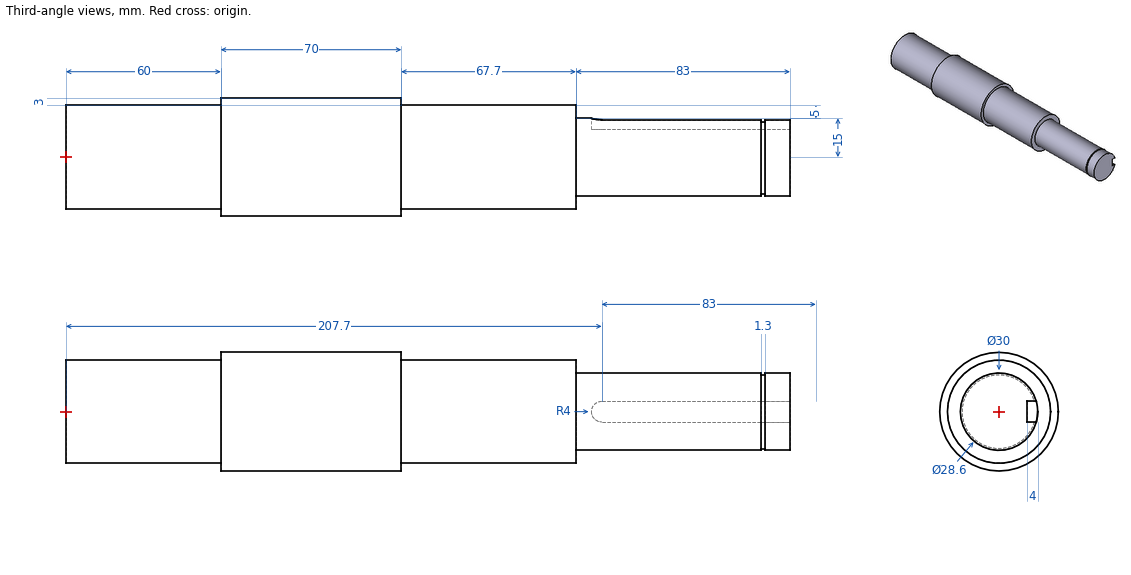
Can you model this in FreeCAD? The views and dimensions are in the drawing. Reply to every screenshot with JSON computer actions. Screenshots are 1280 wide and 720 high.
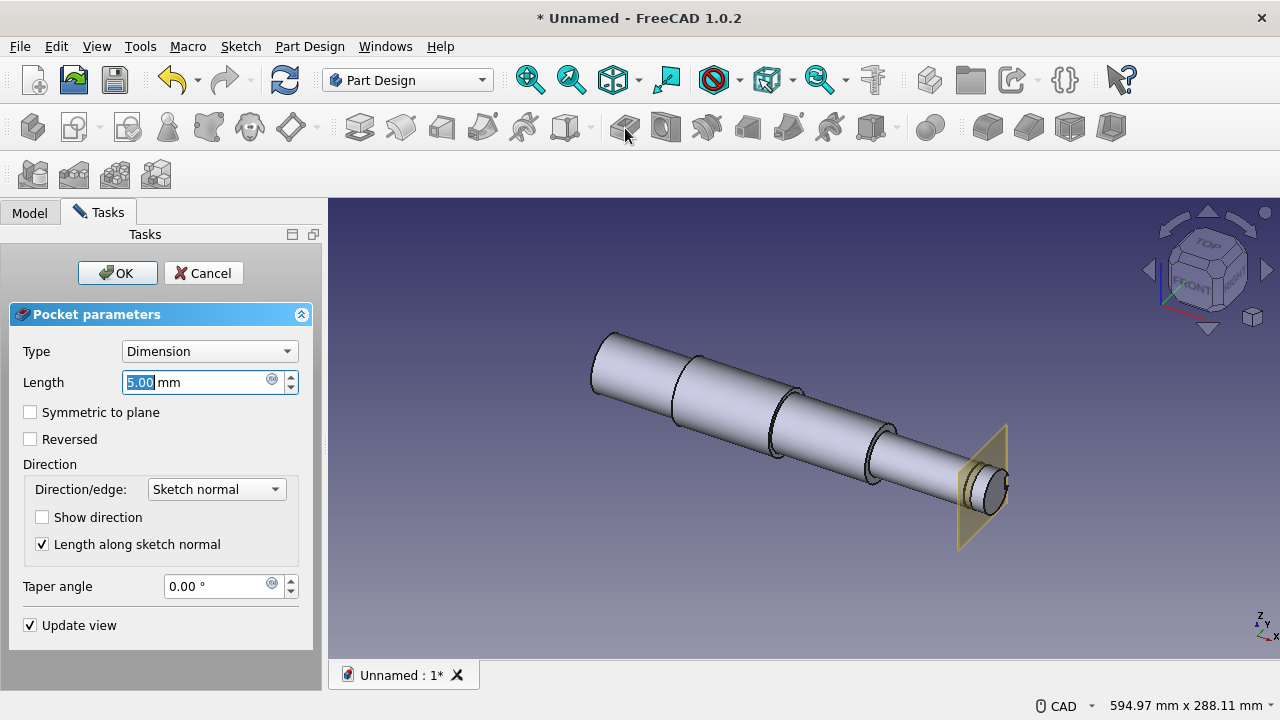
{"action": "type", "text": "1.3"}
{"action": "key", "text": "Tab"}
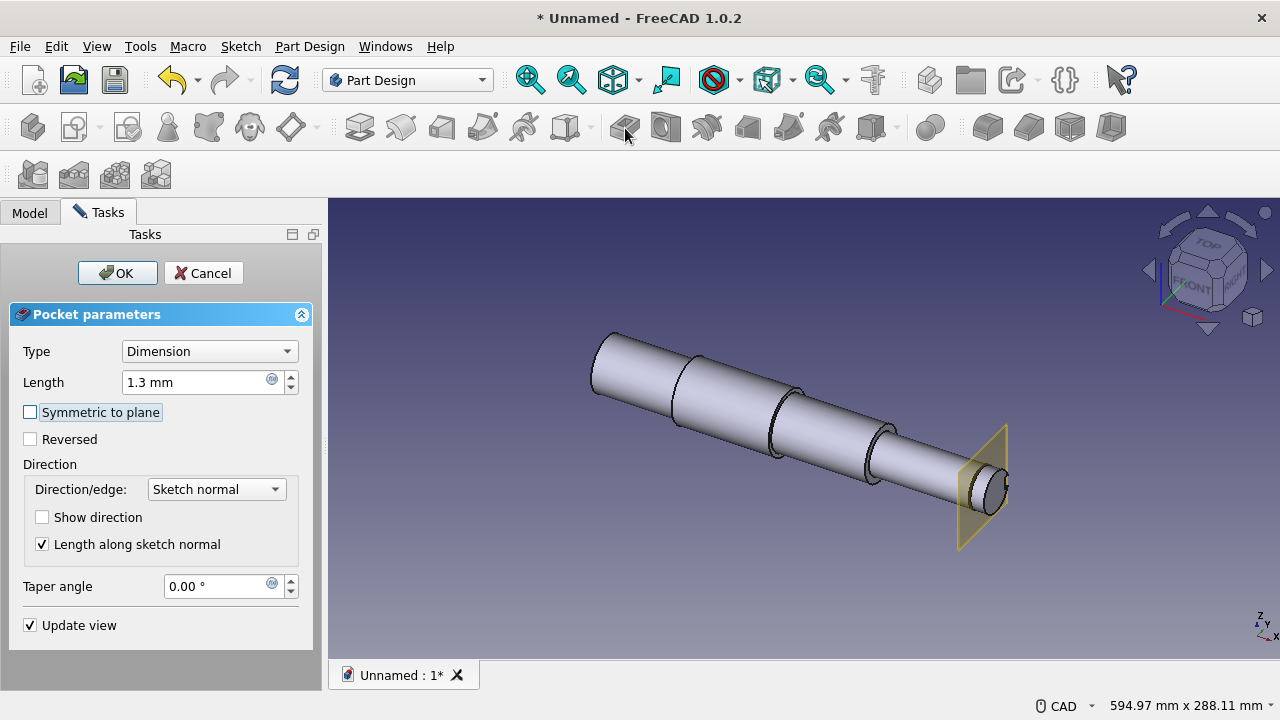
{"action": "left_click", "coordinate": [118, 273]}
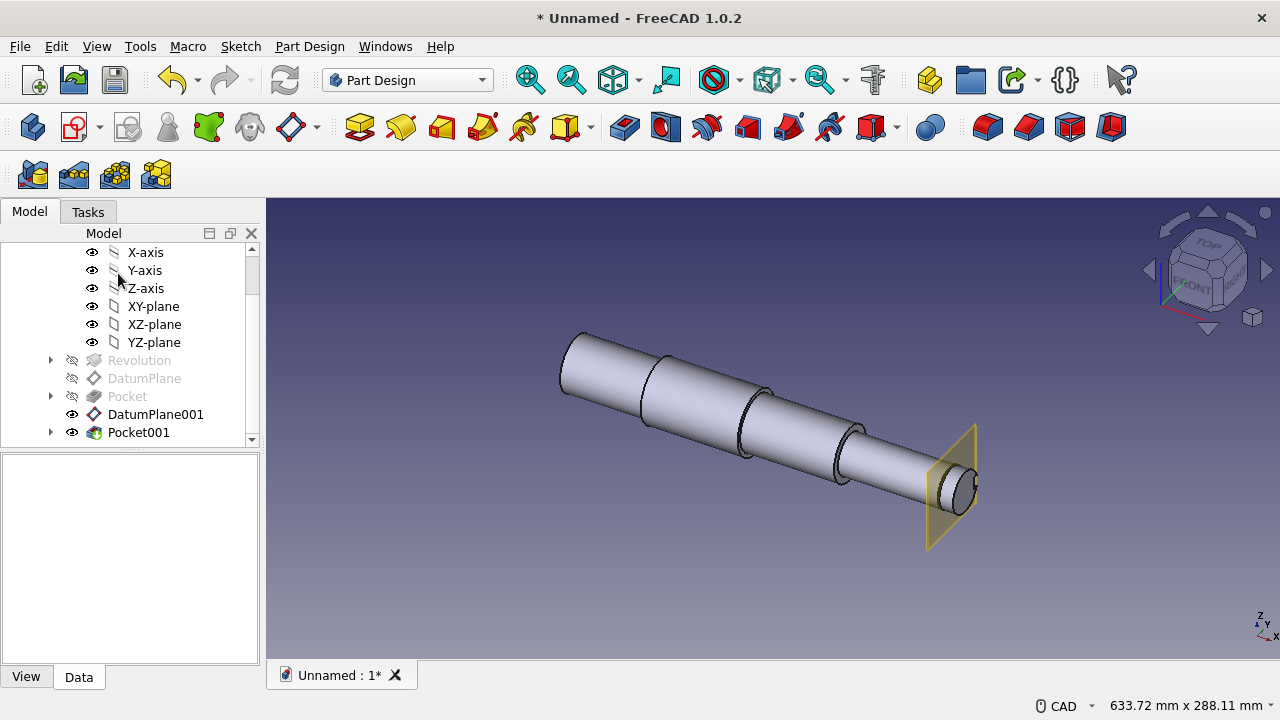
{"action": "left_click", "coordinate": [117, 414]}
{"action": "key", "text": "space"}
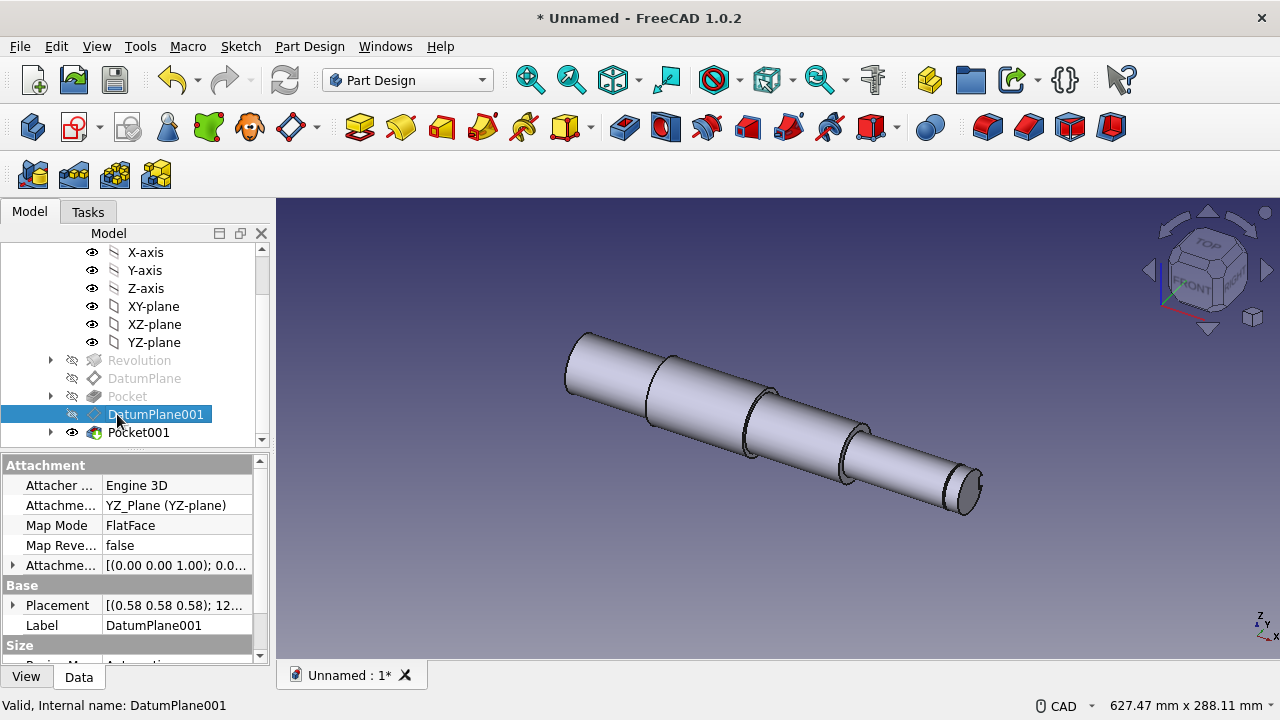
{"action": "key", "text": "0"}